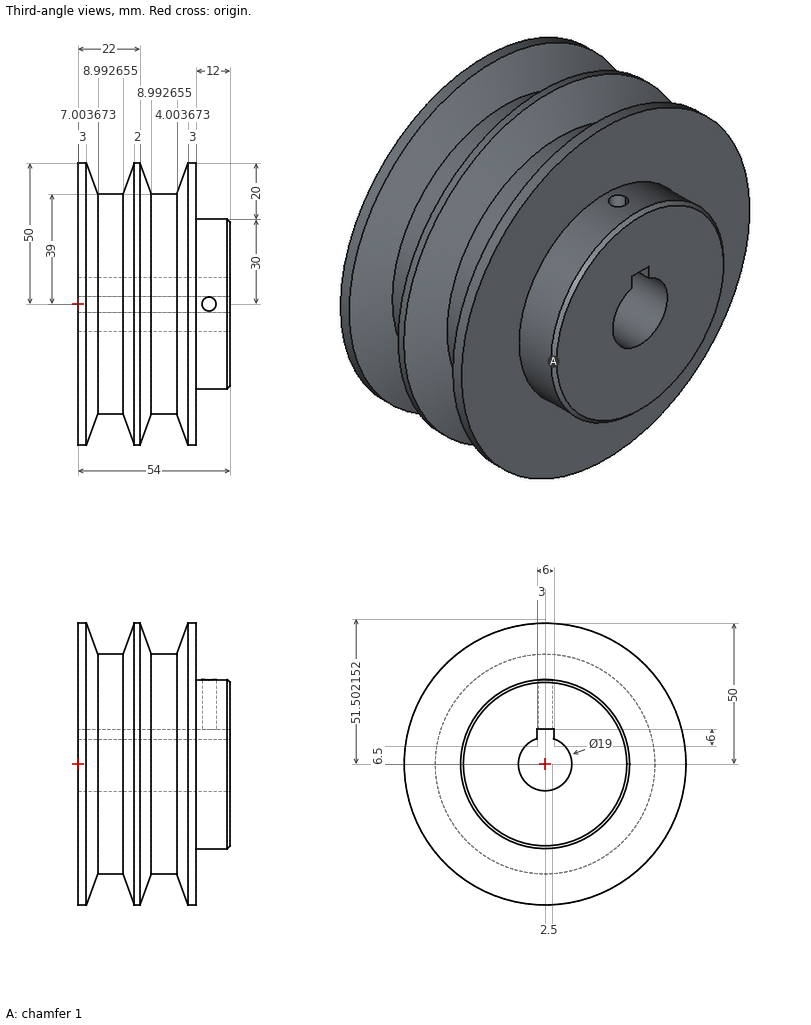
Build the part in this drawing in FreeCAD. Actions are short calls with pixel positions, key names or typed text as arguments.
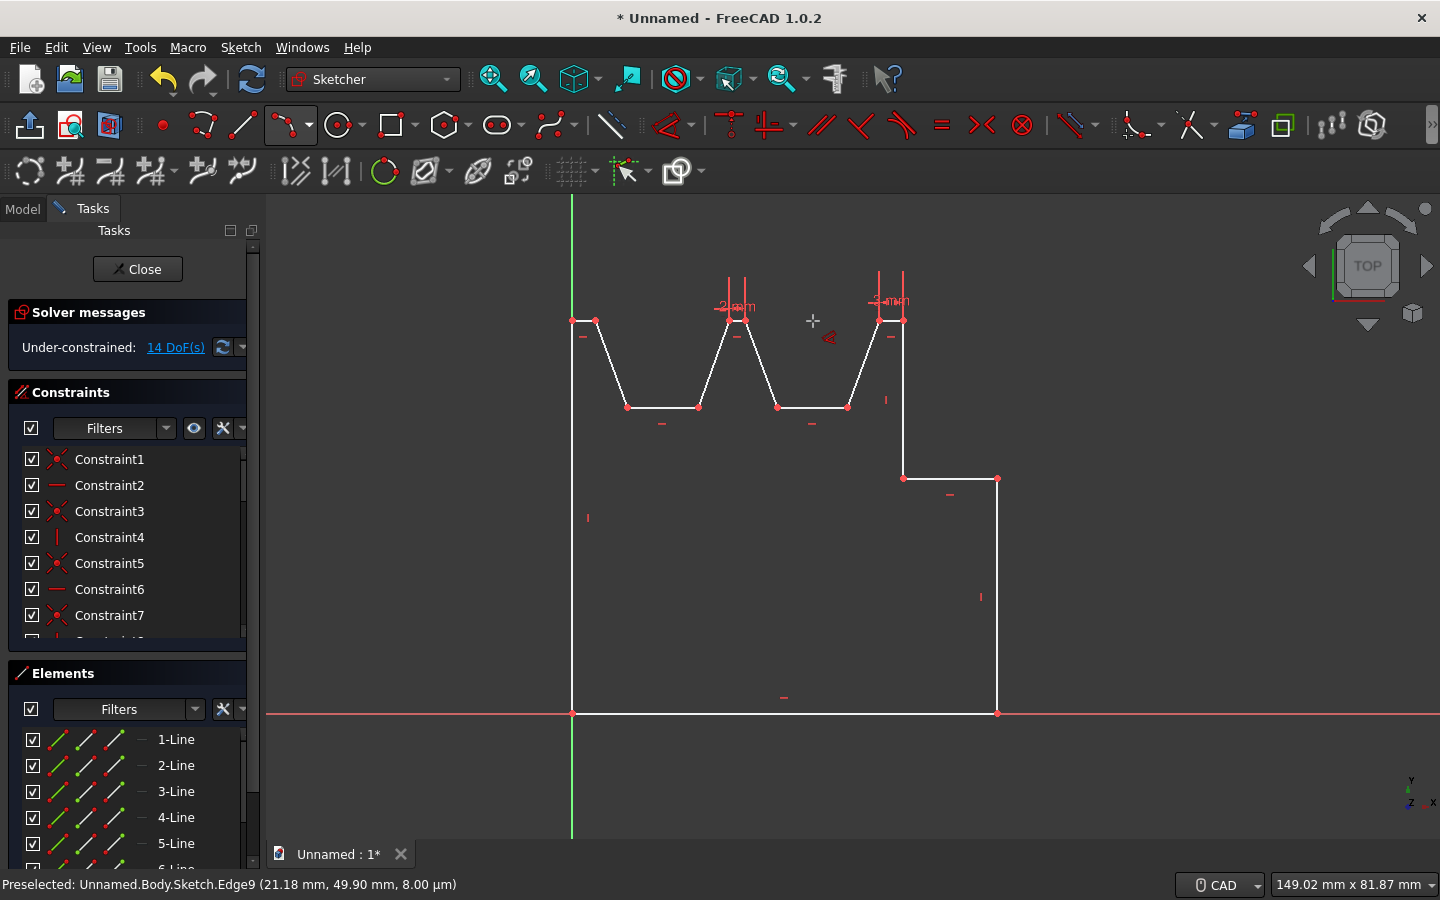
scroll(588, 321, up, 4)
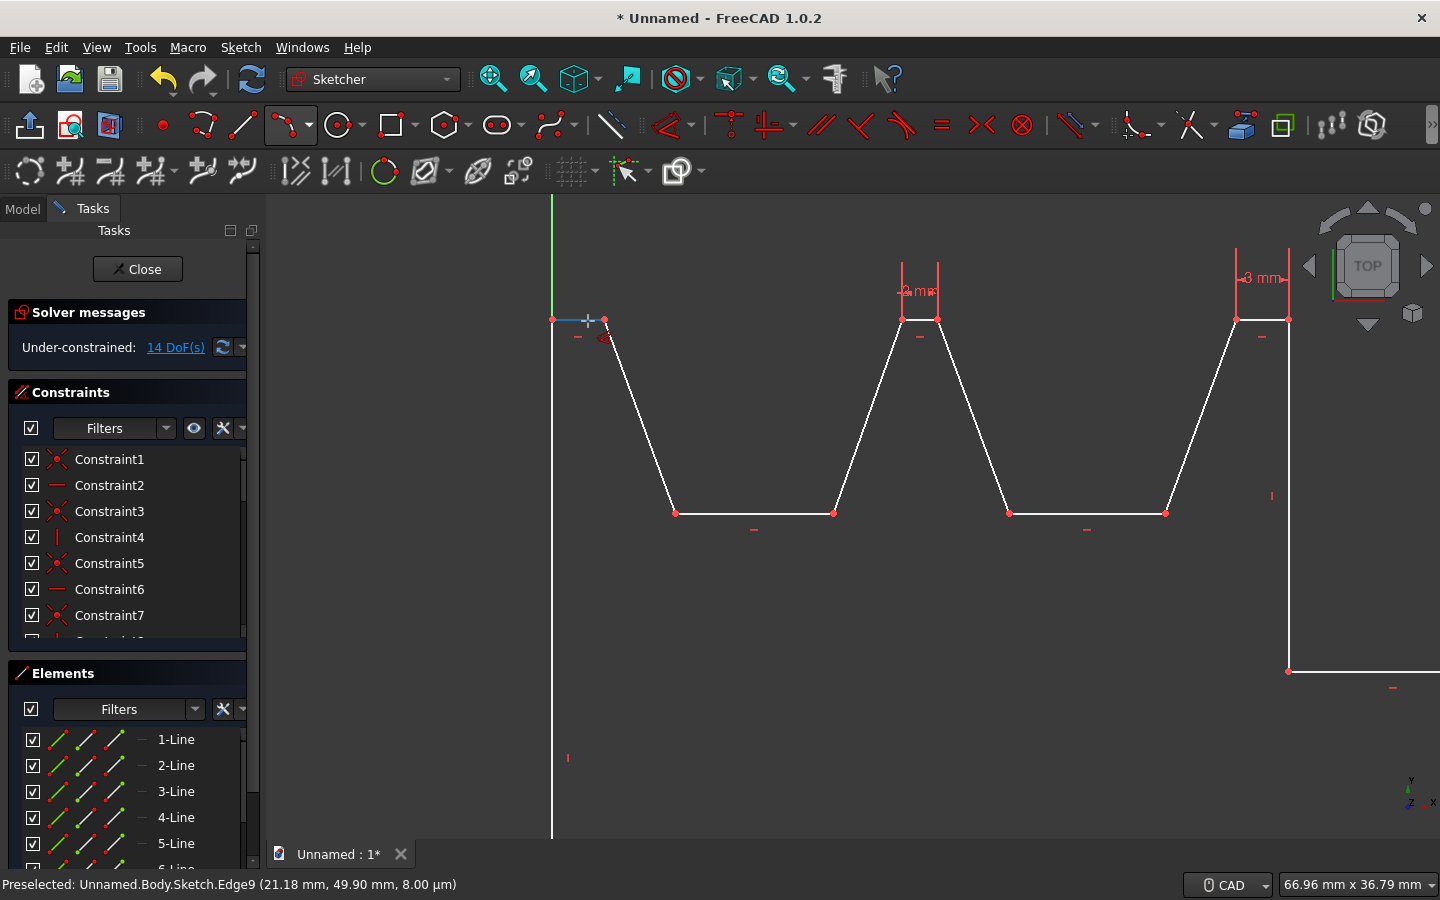
click(589, 320)
click(578, 286)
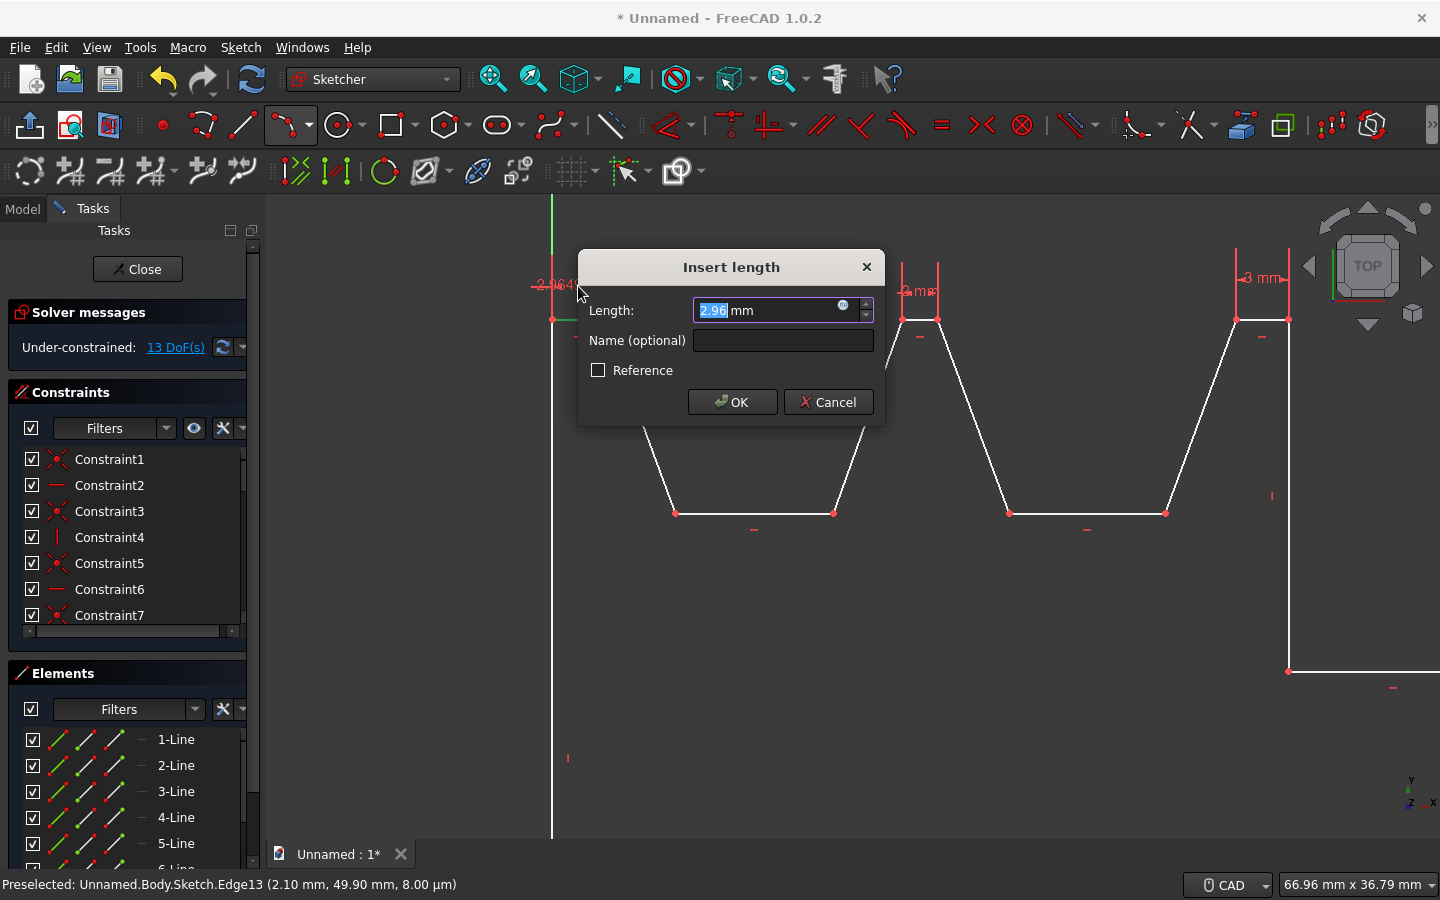
text(3)
key(Return)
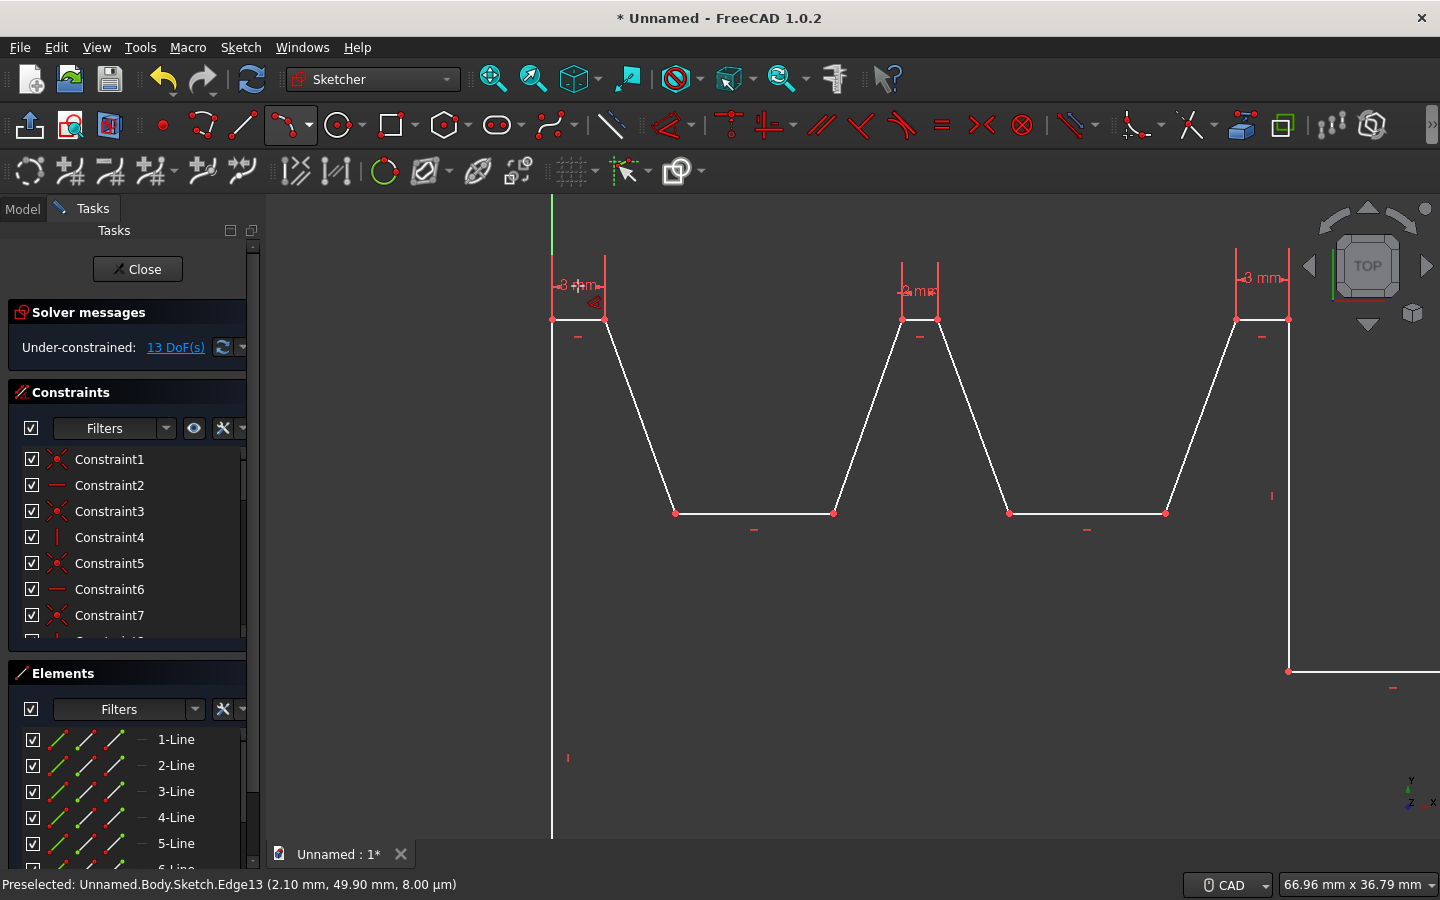
scroll(588, 321, down, 4)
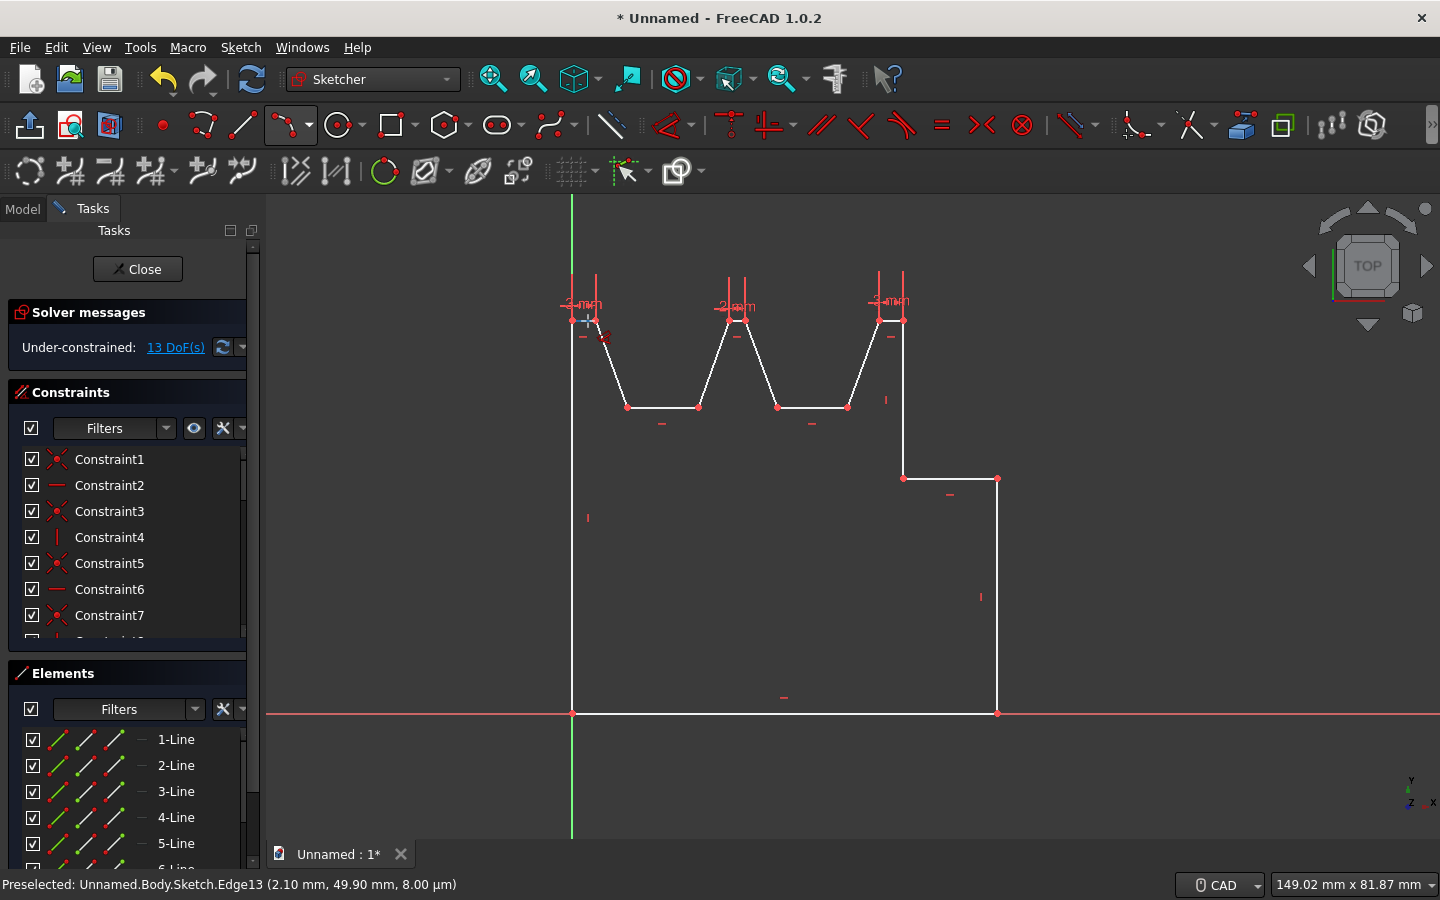
click(700, 714)
click(785, 748)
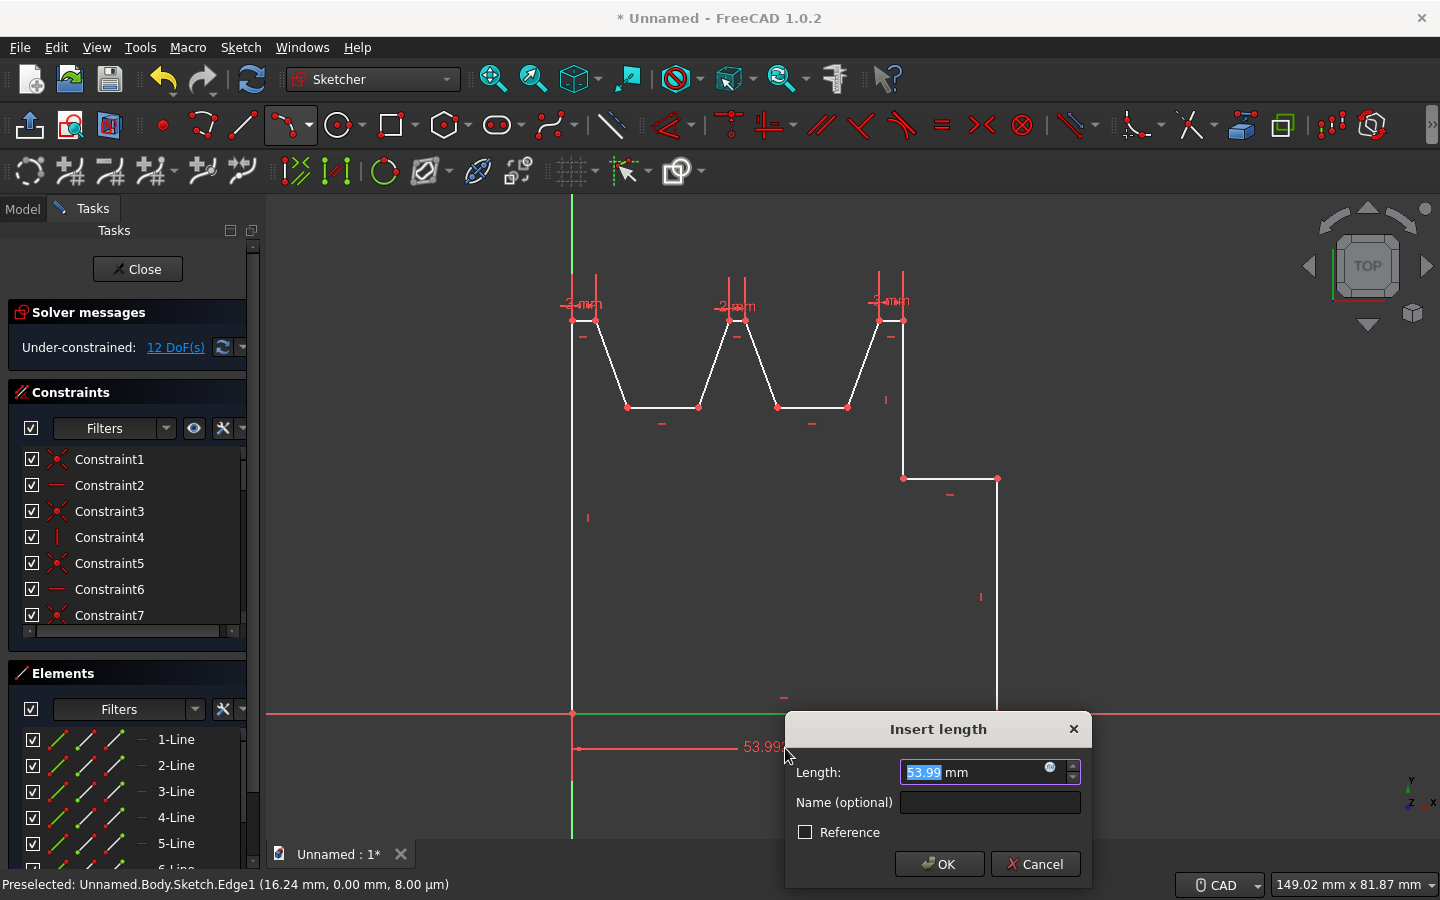
text(54)
key(Return)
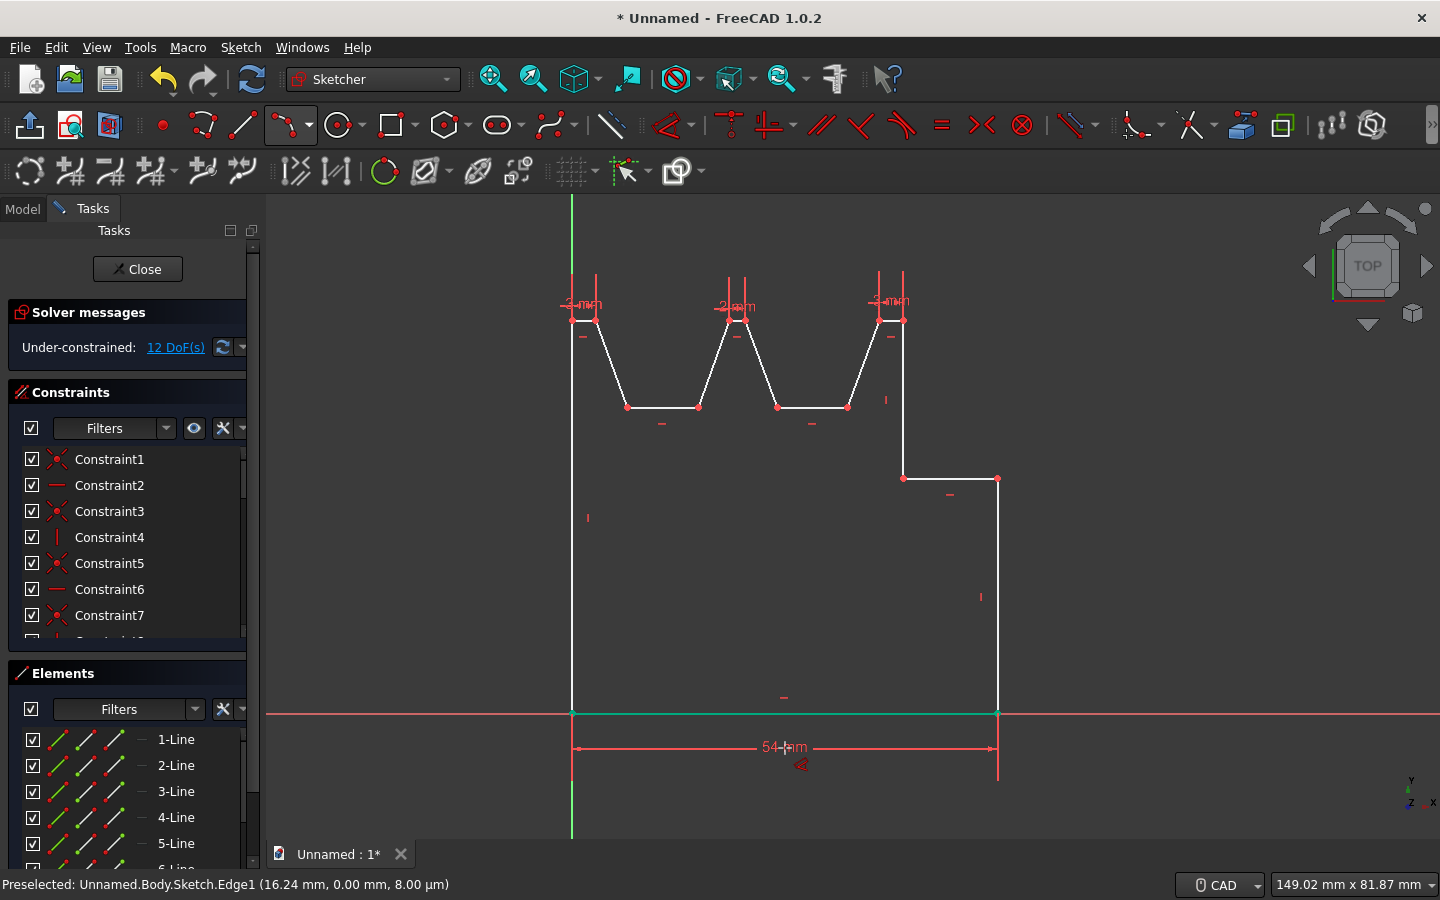
click(998, 643)
click(1032, 596)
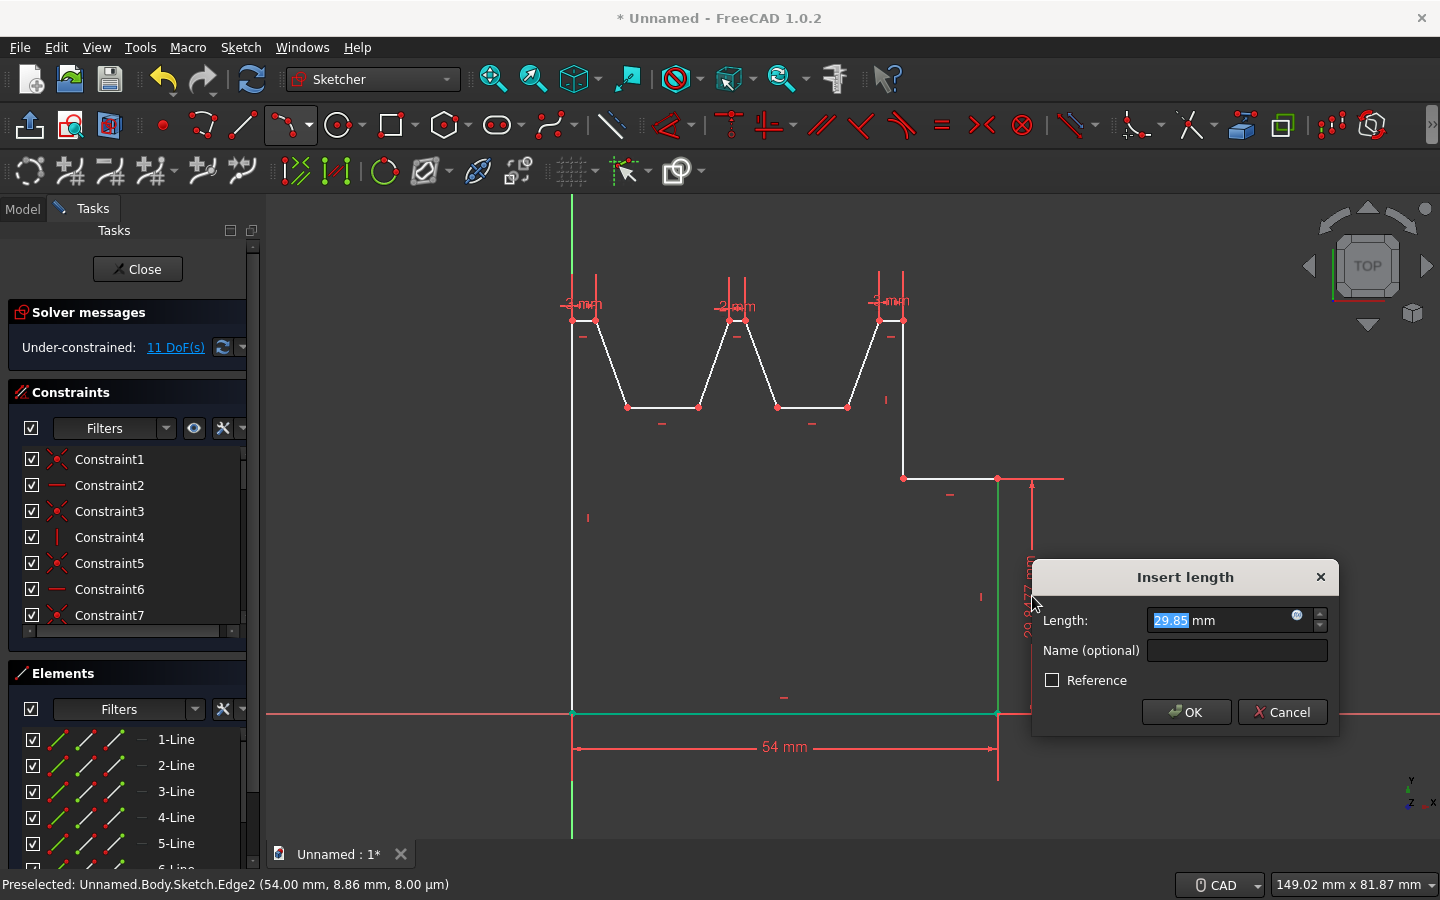
text(30)
key(Return)